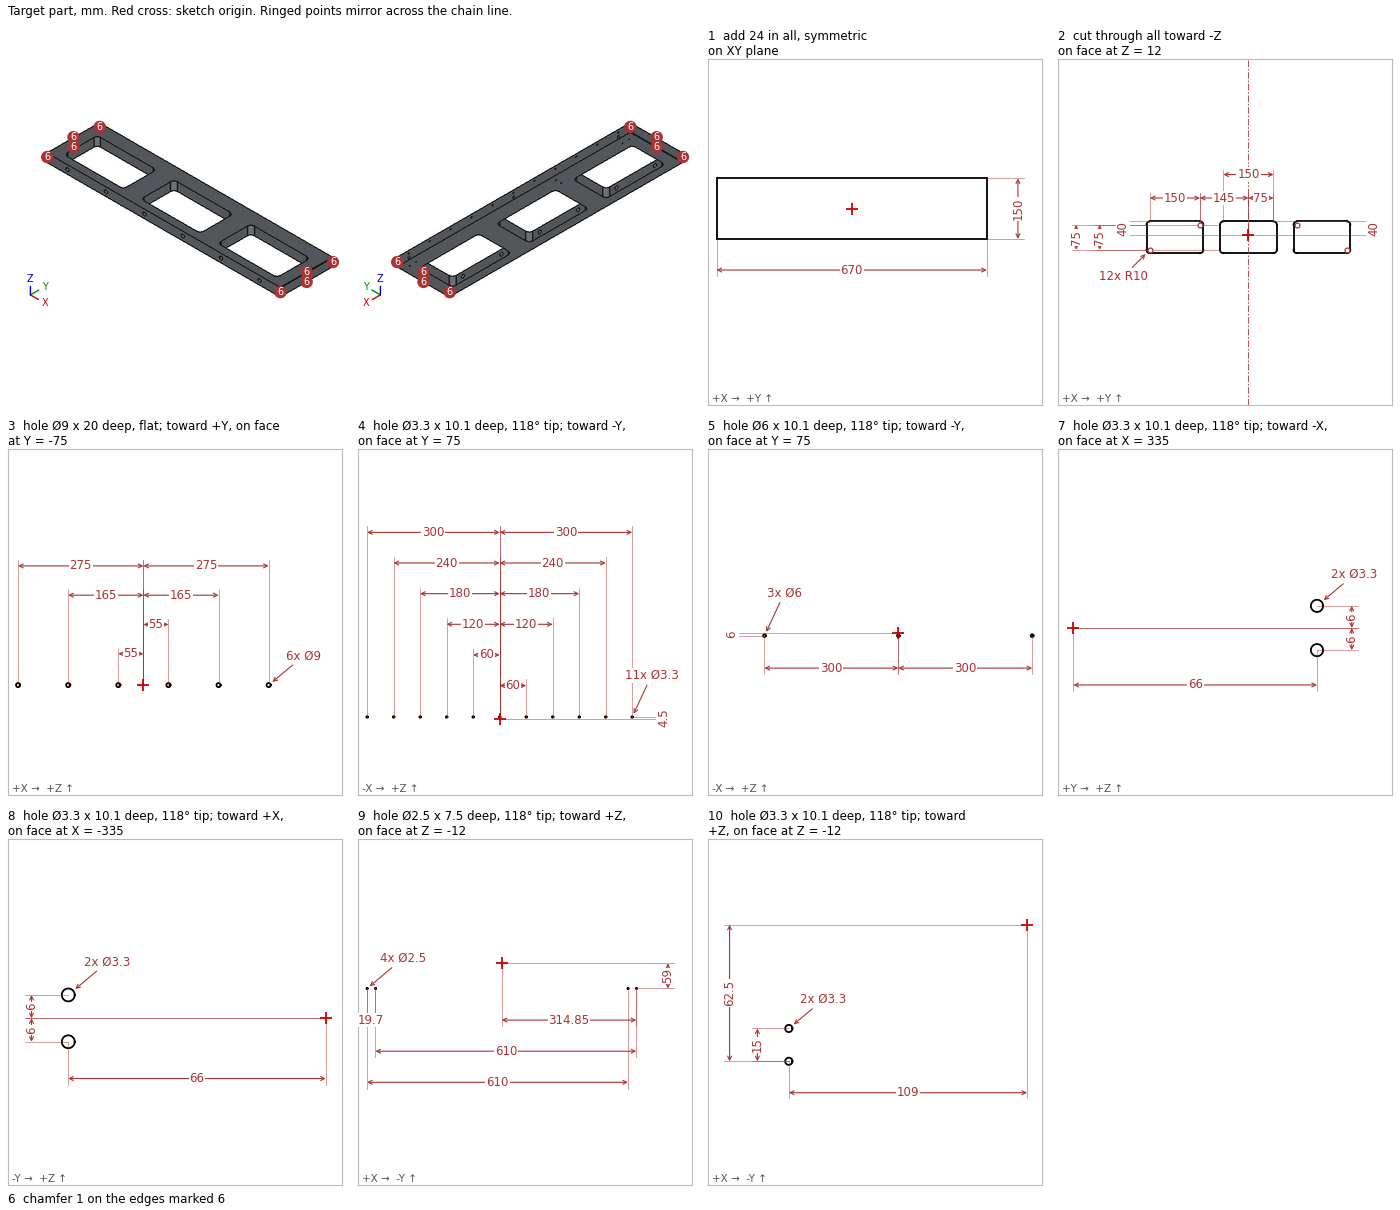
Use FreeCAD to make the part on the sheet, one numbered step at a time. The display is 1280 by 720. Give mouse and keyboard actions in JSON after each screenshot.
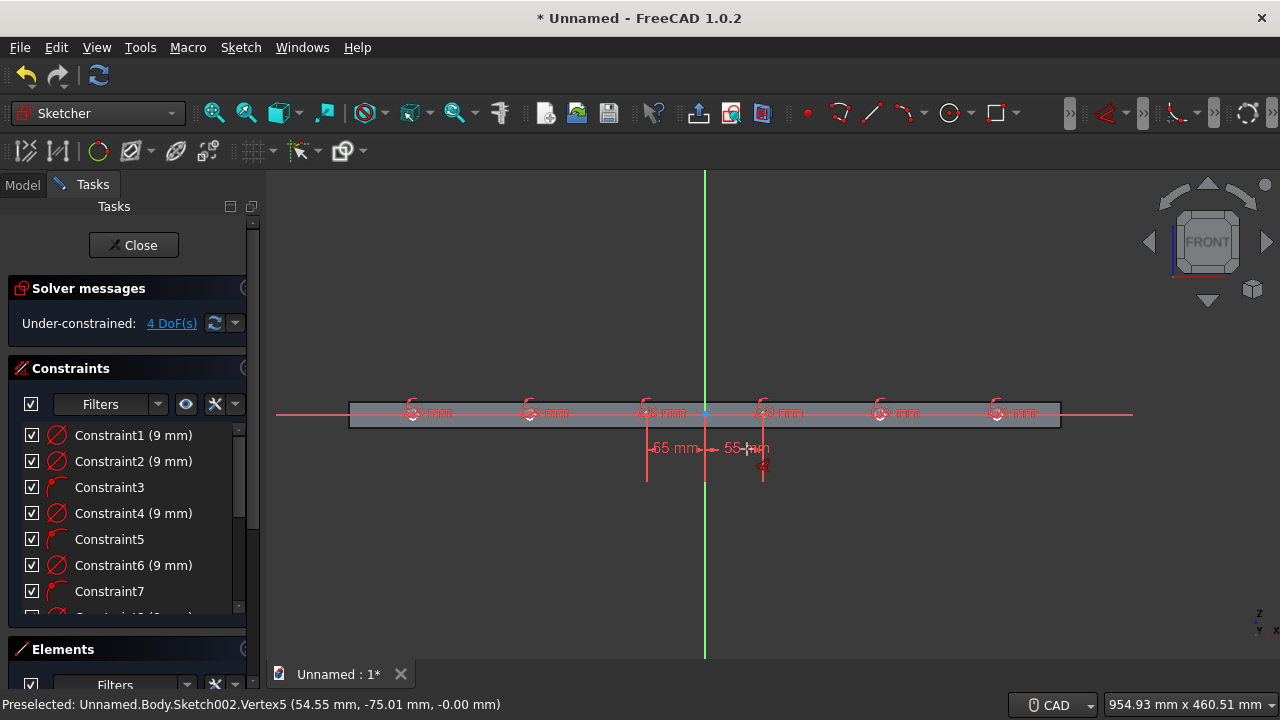
{"action": "left_click", "coordinate": [997, 415]}
{"action": "left_click", "coordinate": [851, 449]}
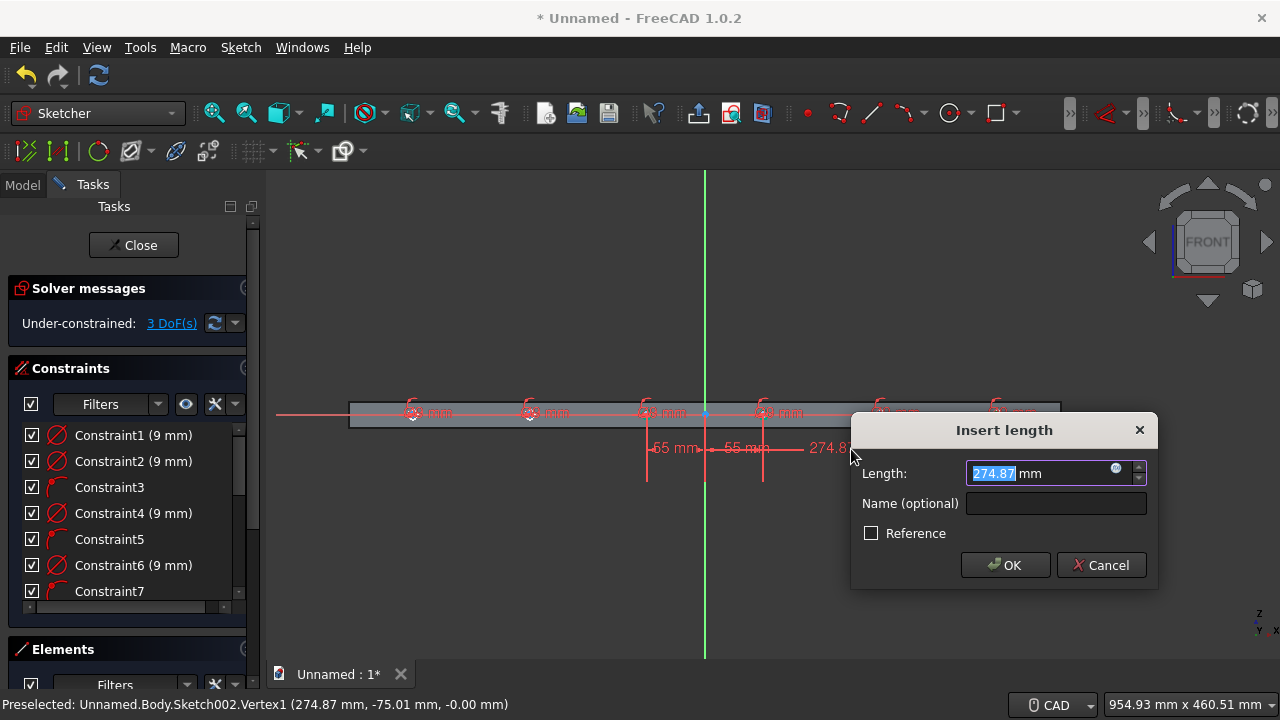
{"action": "type", "text": "275"}
{"action": "key", "text": "Return"}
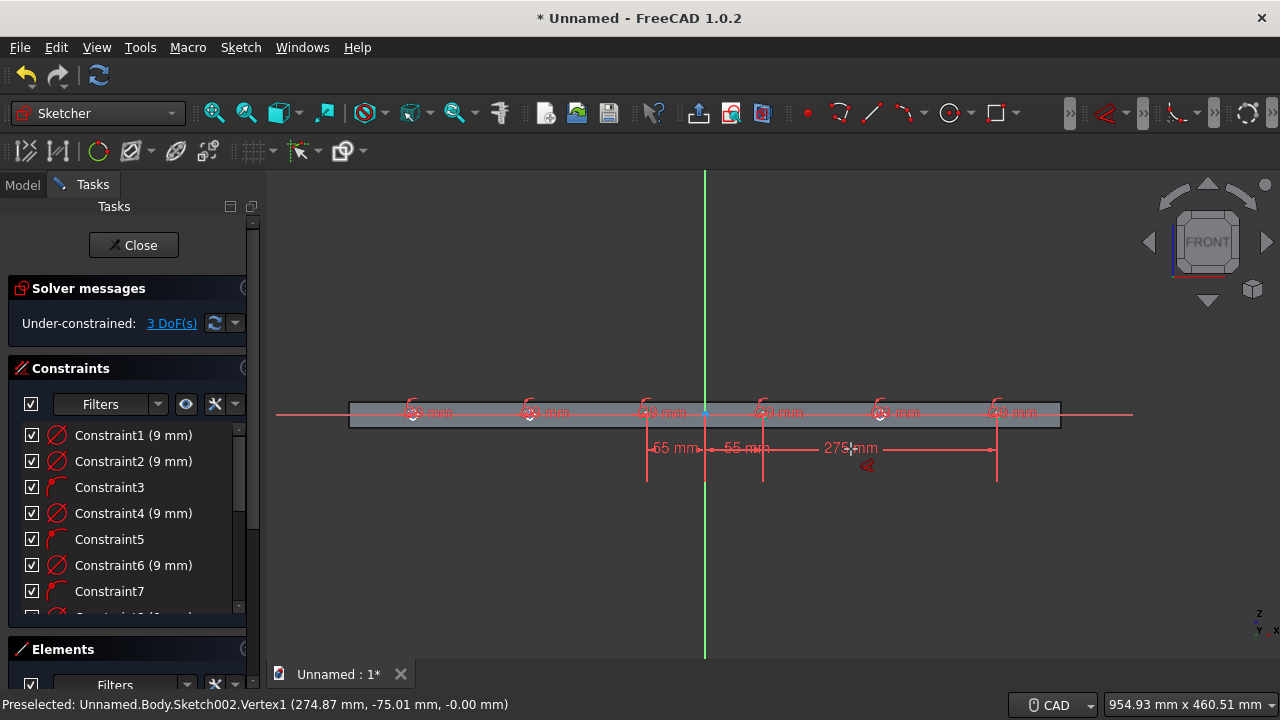
{"action": "left_click", "coordinate": [413, 415]}
{"action": "left_click", "coordinate": [559, 449]}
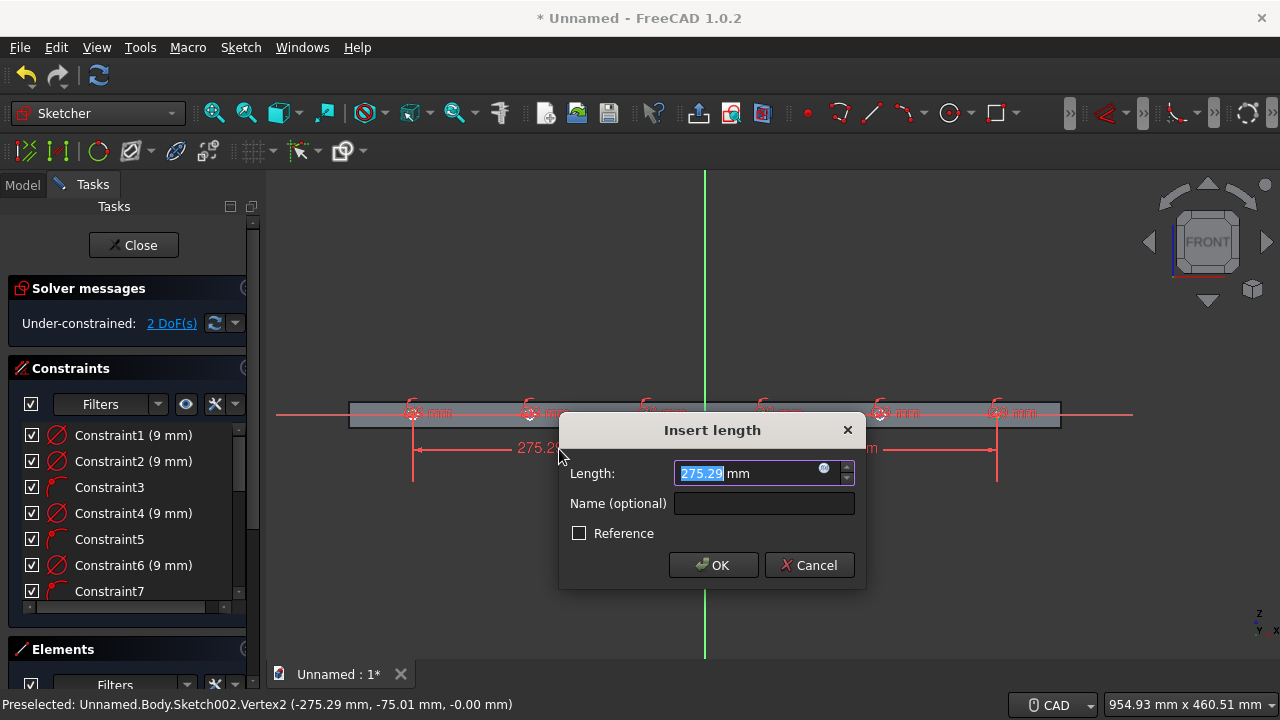
{"action": "type", "text": "275"}
{"action": "key", "text": "Return"}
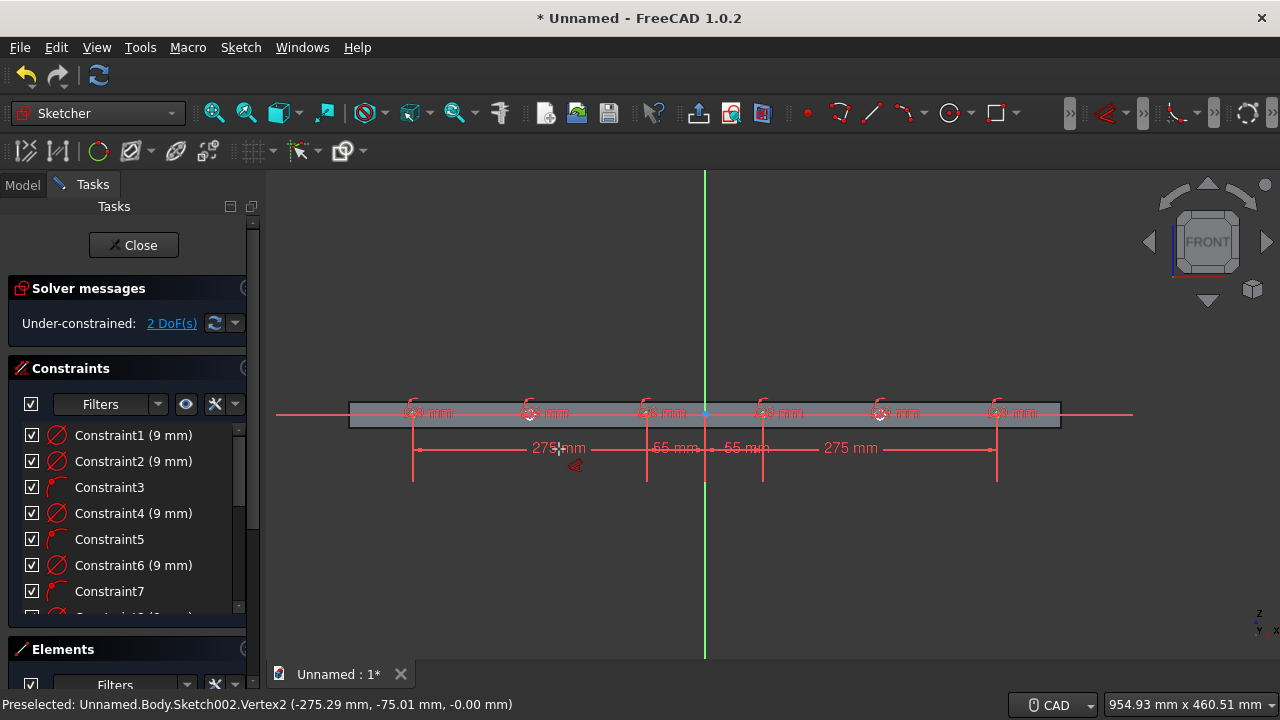
{"action": "left_click", "coordinate": [530, 415]}
{"action": "left_click", "coordinate": [617, 381]}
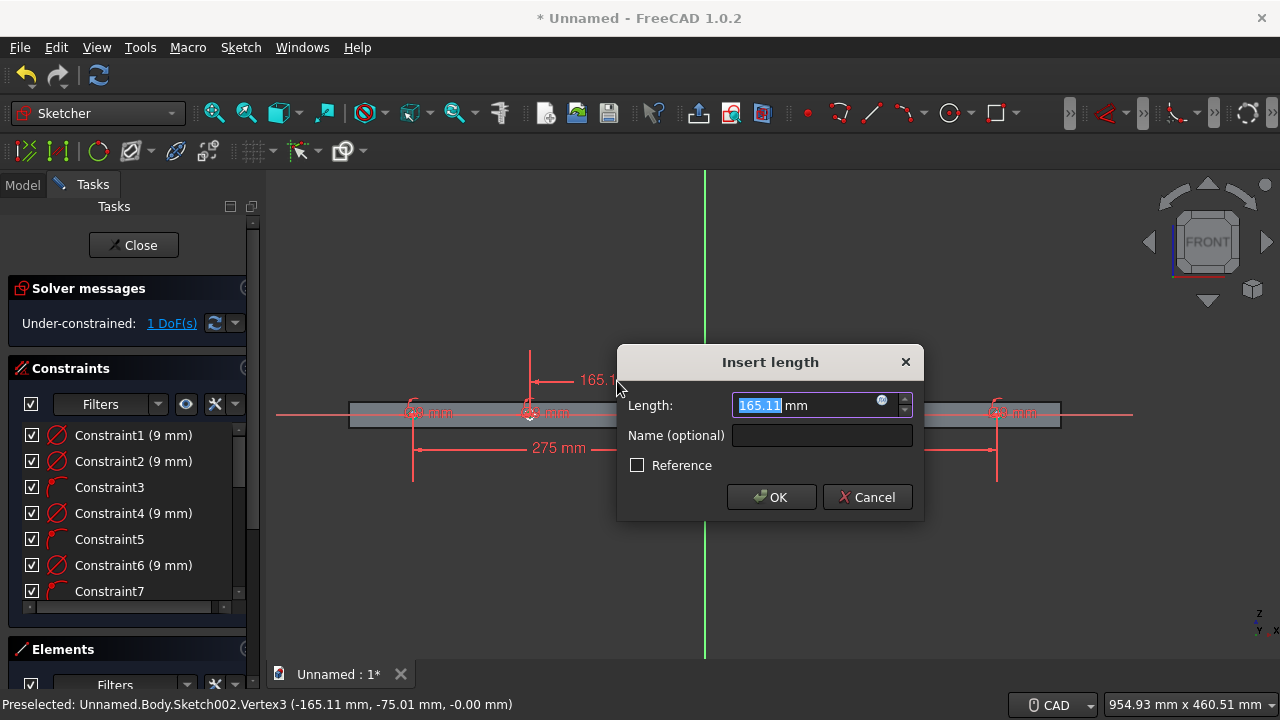
{"action": "type", "text": "165"}
{"action": "key", "text": "Return"}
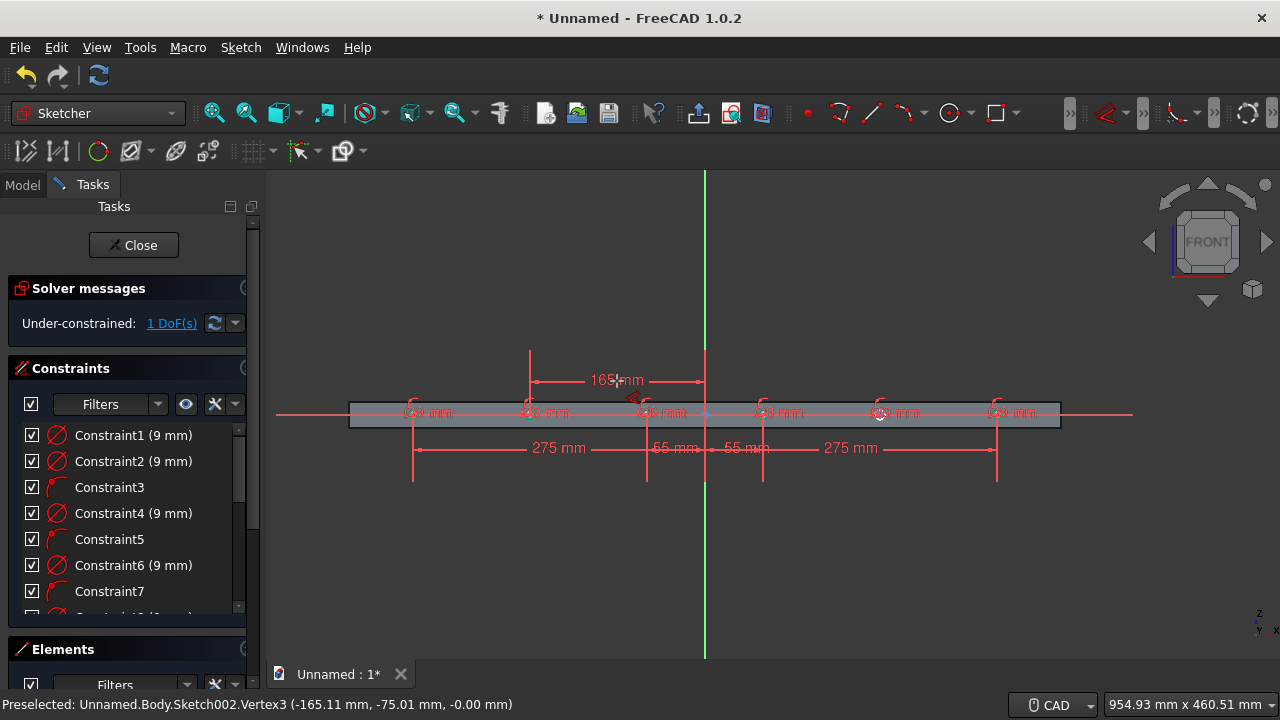
{"action": "left_click", "coordinate": [880, 415]}
{"action": "left_click", "coordinate": [793, 381]}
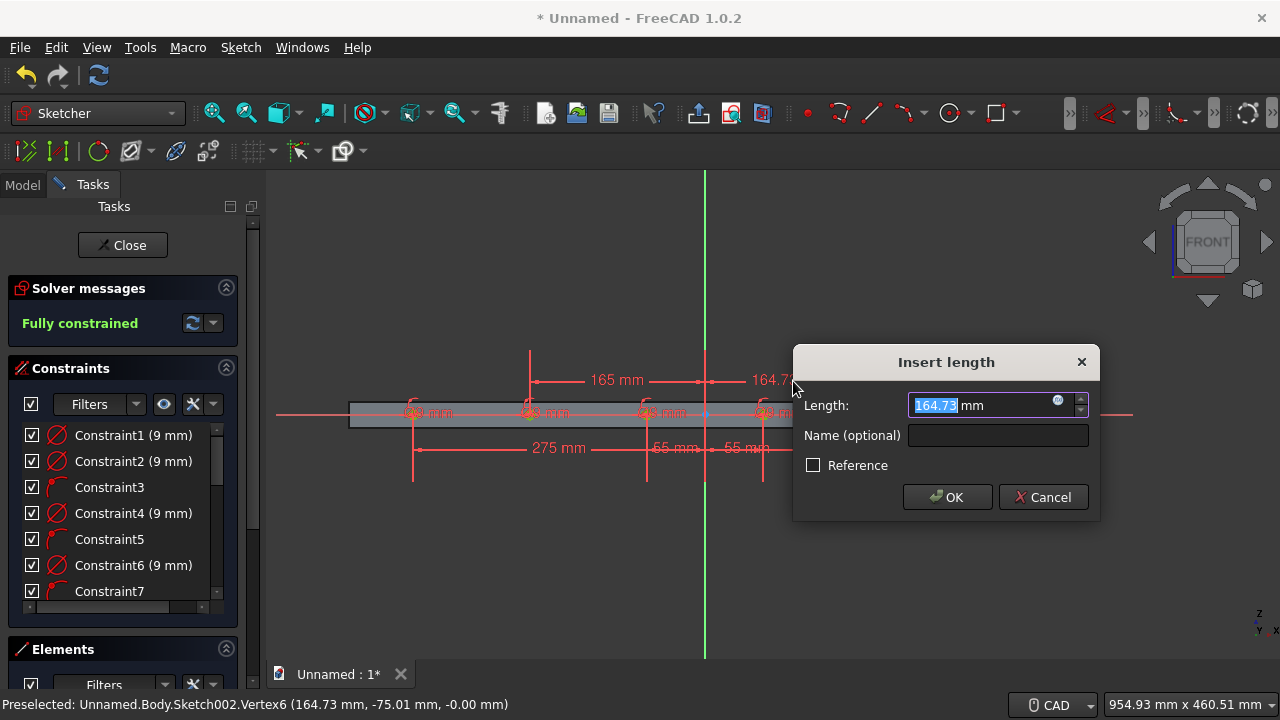
{"action": "type", "text": "165"}
{"action": "key", "text": "Return"}
{"action": "key", "text": "Escape"}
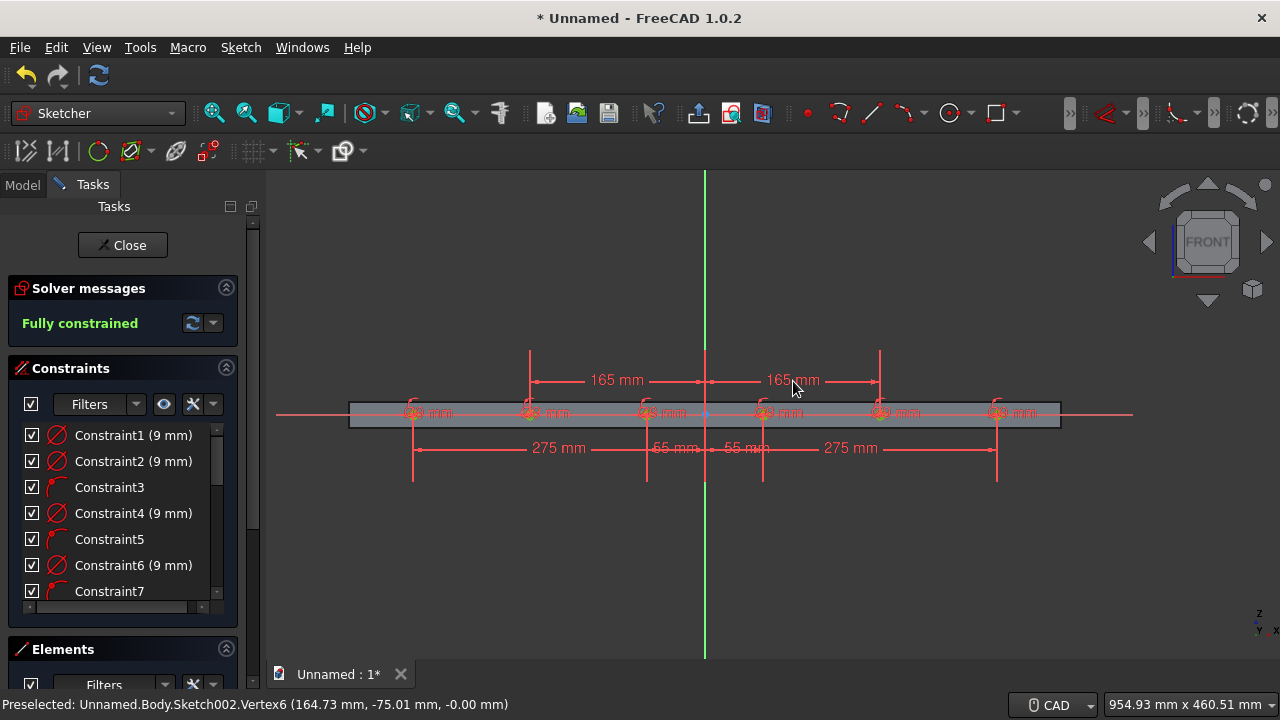
{"action": "left_click", "coordinate": [123, 245]}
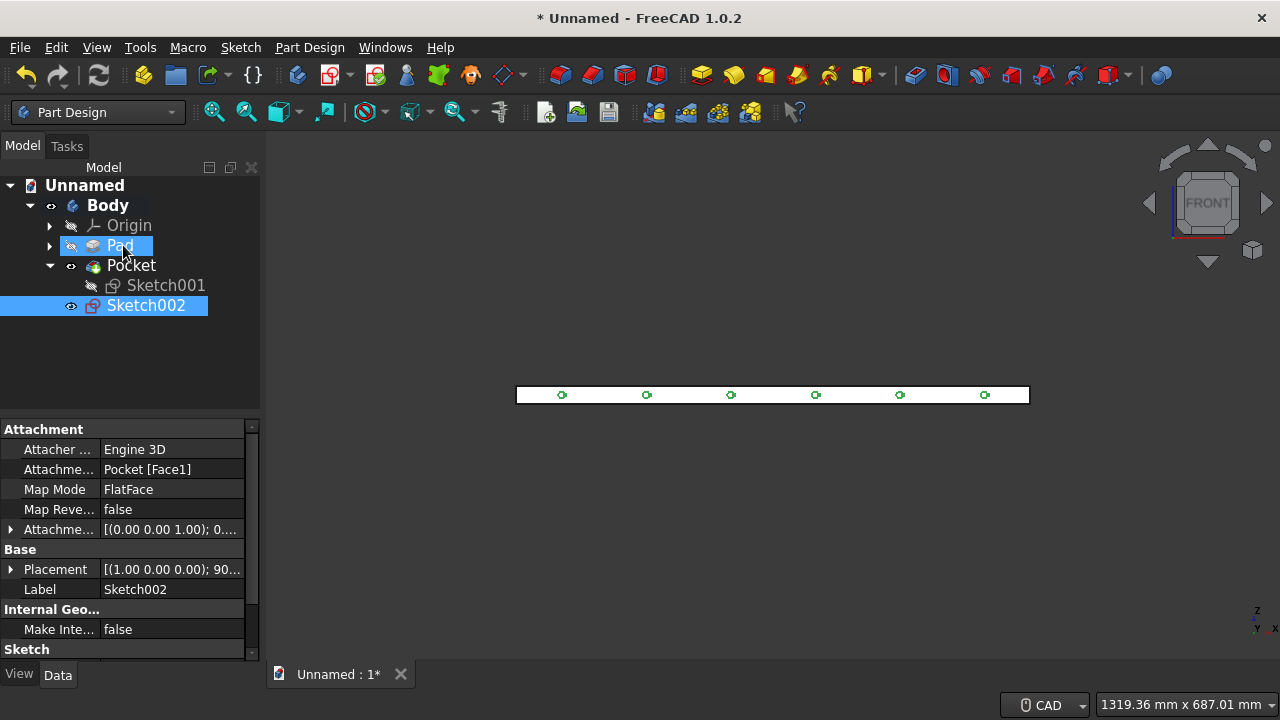
{"action": "left_click", "coordinate": [948, 76]}